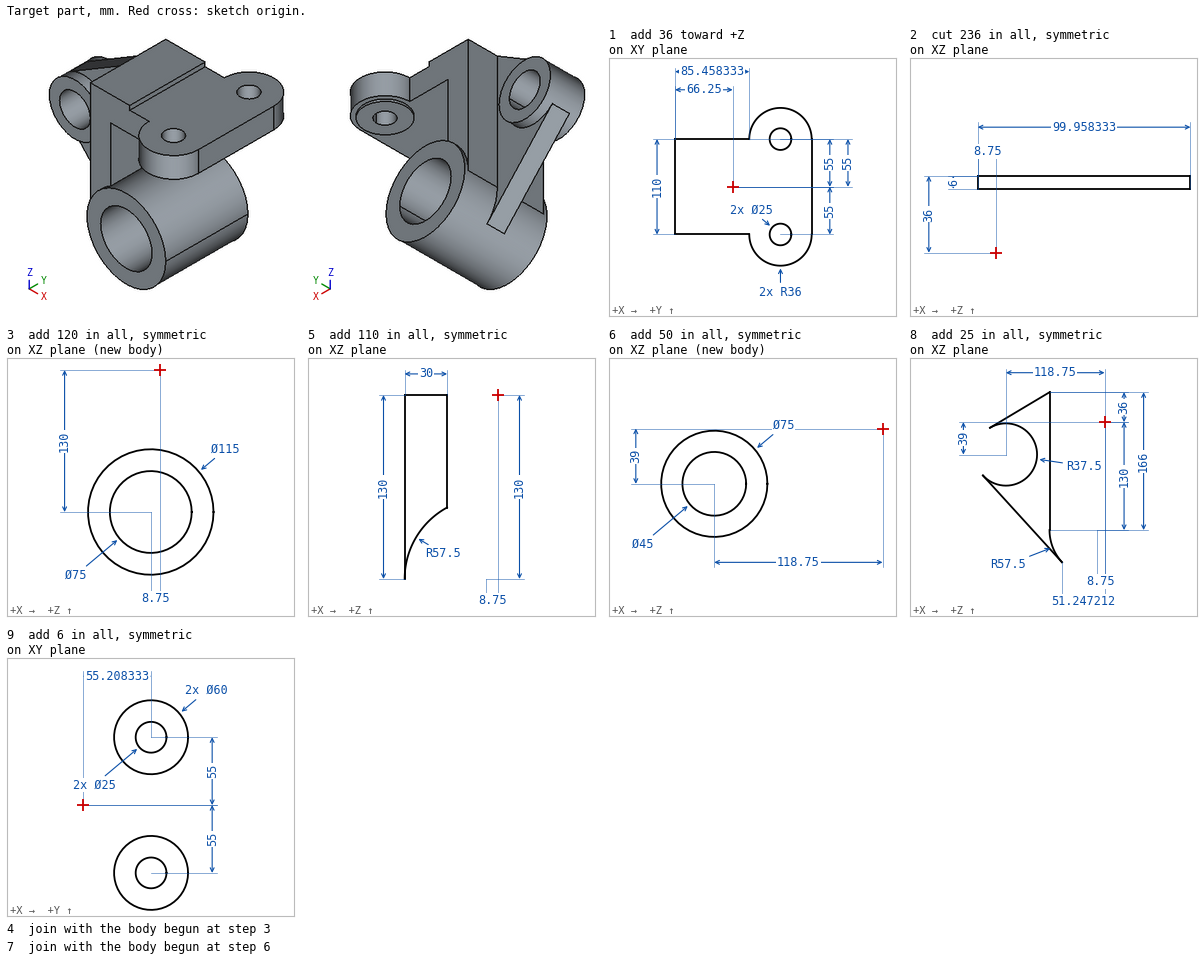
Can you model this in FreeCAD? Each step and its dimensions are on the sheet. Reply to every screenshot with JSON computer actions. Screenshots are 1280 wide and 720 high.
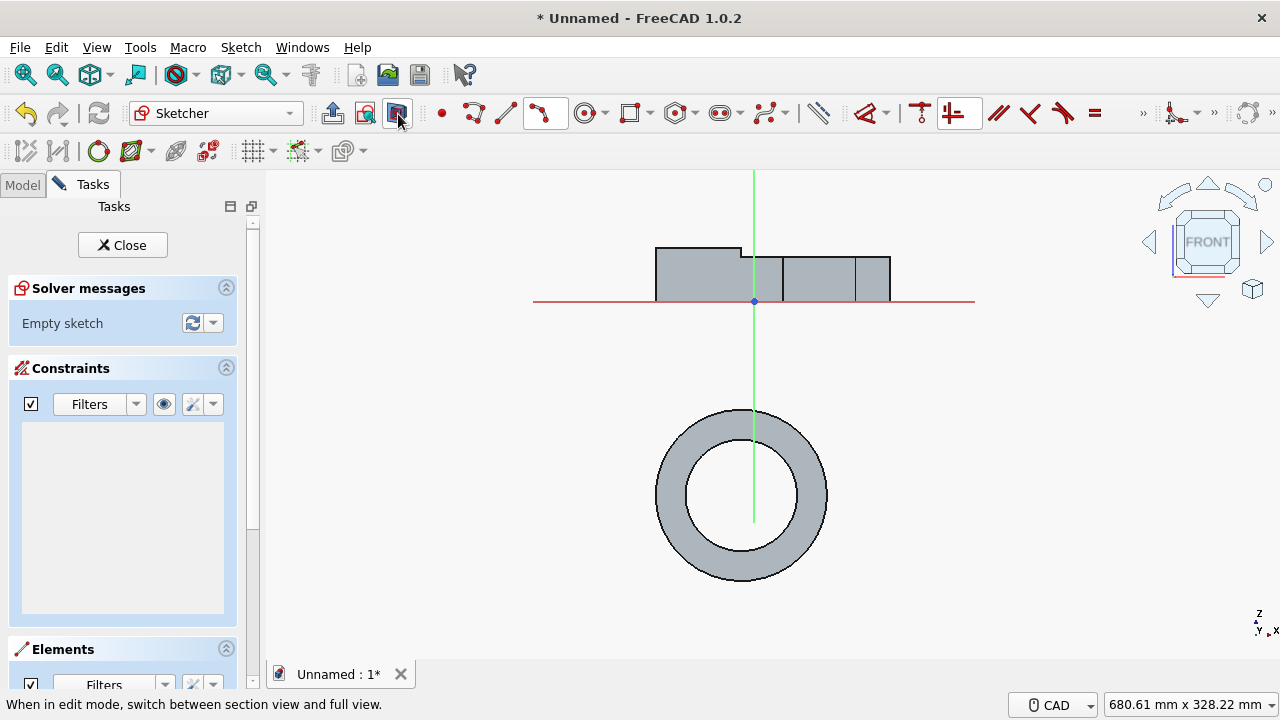
{"action": "scroll", "coordinate": [706, 366], "scroll_direction": "up", "scroll_amount": 2}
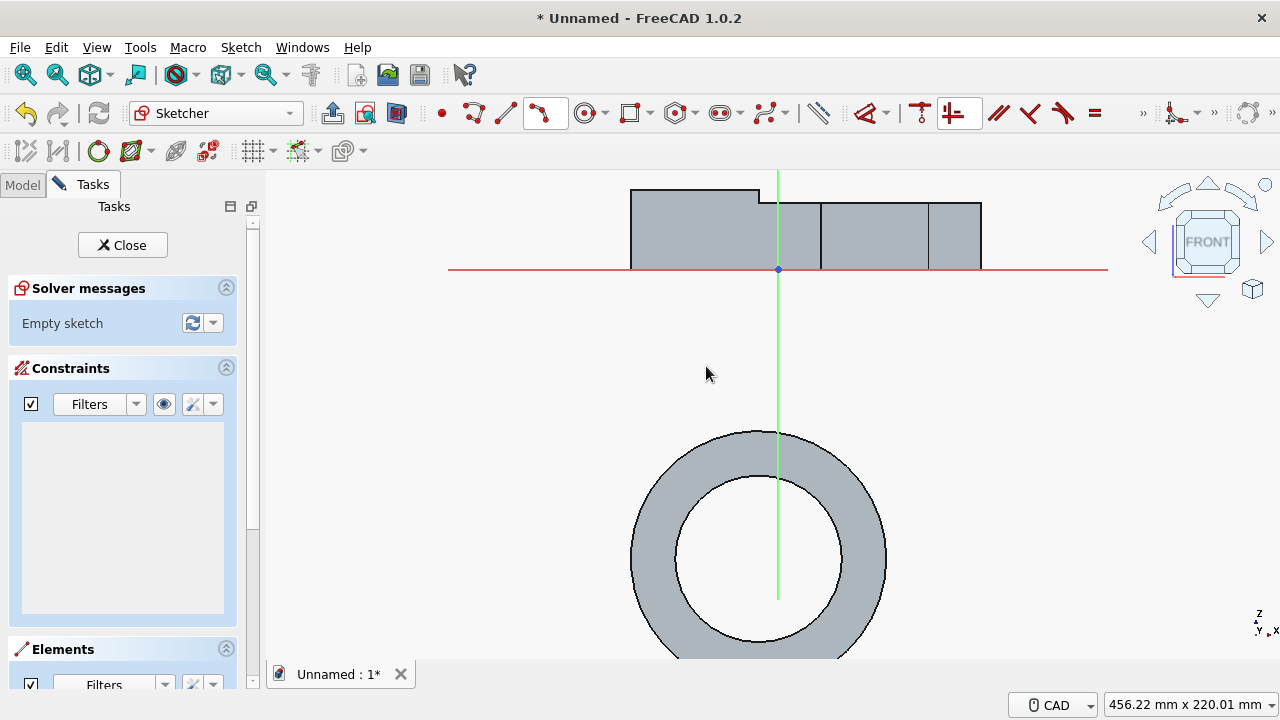
{"action": "left_click", "coordinate": [474, 114]}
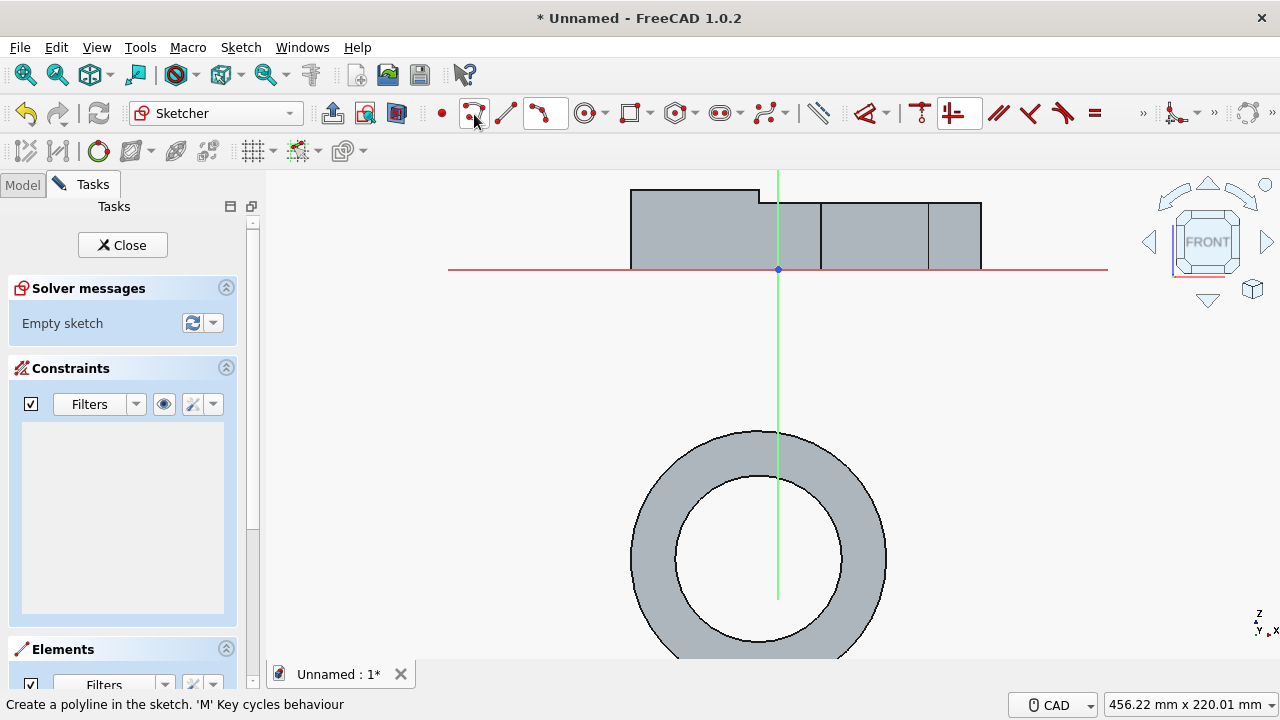
{"action": "left_click", "coordinate": [631, 559]}
{"action": "left_click", "coordinate": [631, 270]}
{"action": "left_click", "coordinate": [697, 279]}
{"action": "left_click", "coordinate": [697, 447]}
{"action": "right_click", "coordinate": [697, 447]}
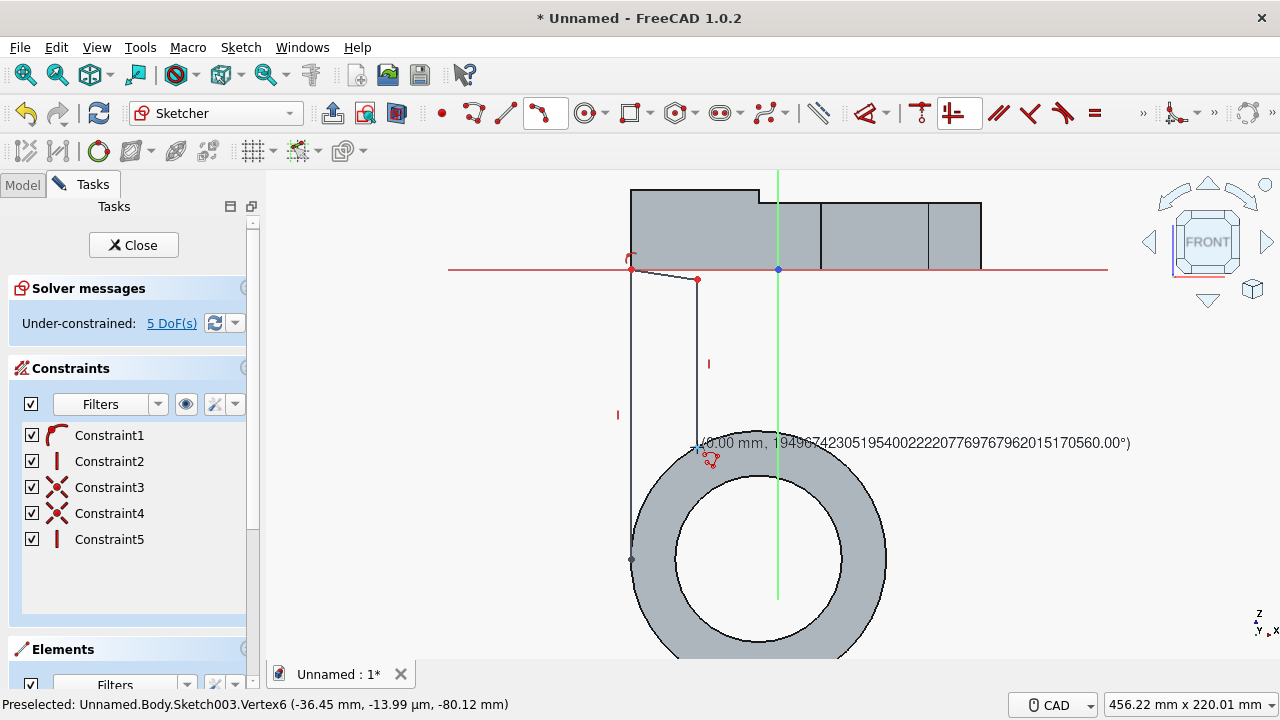
{"action": "left_click", "coordinate": [540, 114]}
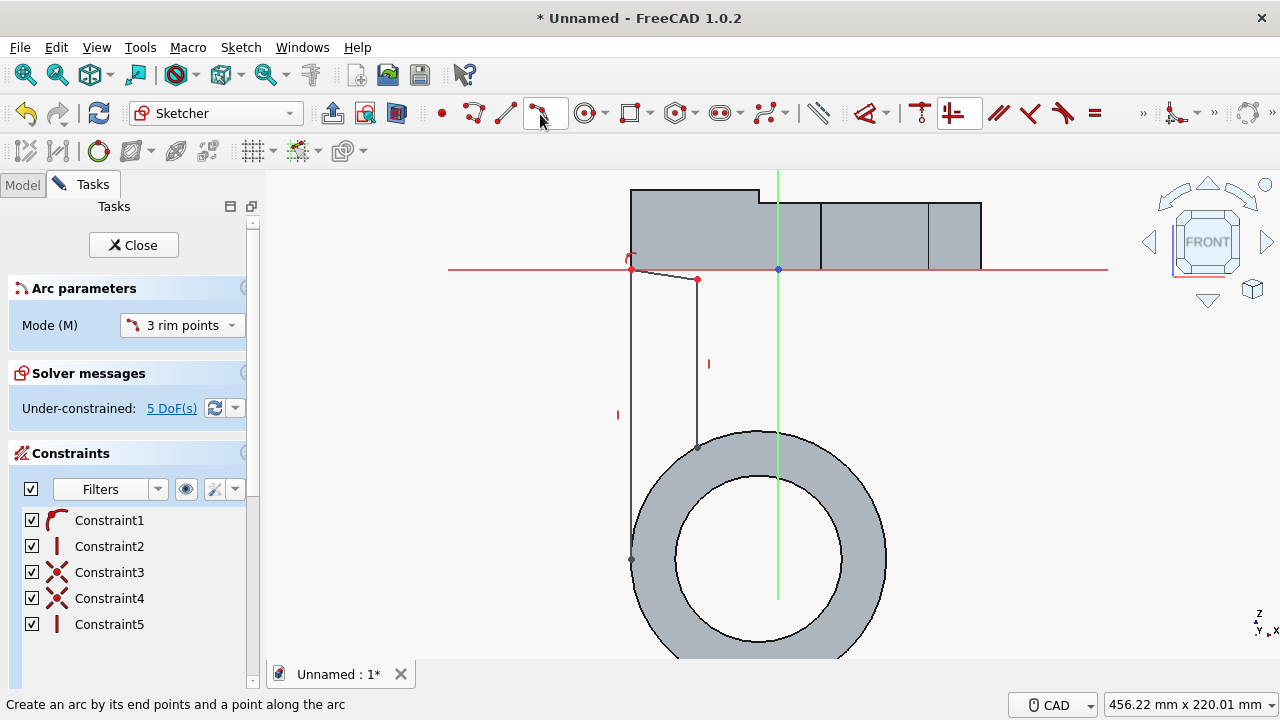
{"action": "left_click", "coordinate": [697, 448]}
{"action": "left_click", "coordinate": [631, 560]}
{"action": "left_click", "coordinate": [649, 494]}
{"action": "key", "text": "Escape"}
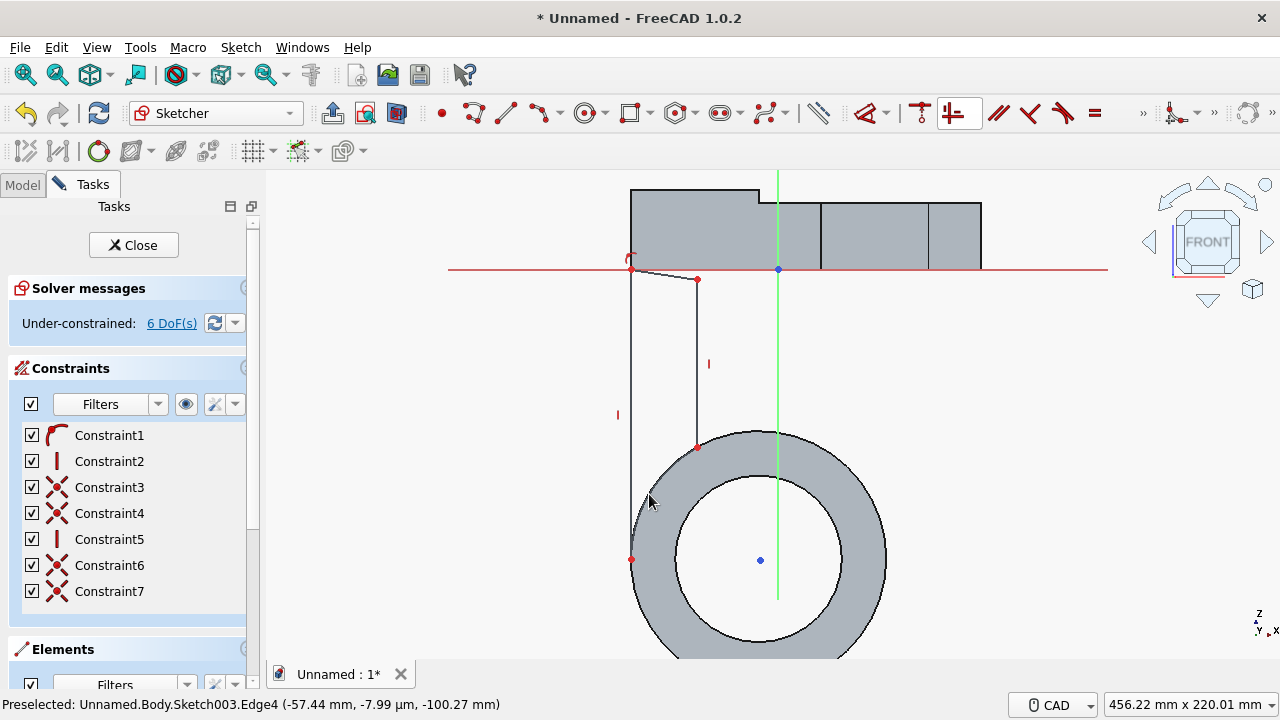
{"action": "left_click", "coordinate": [651, 273]}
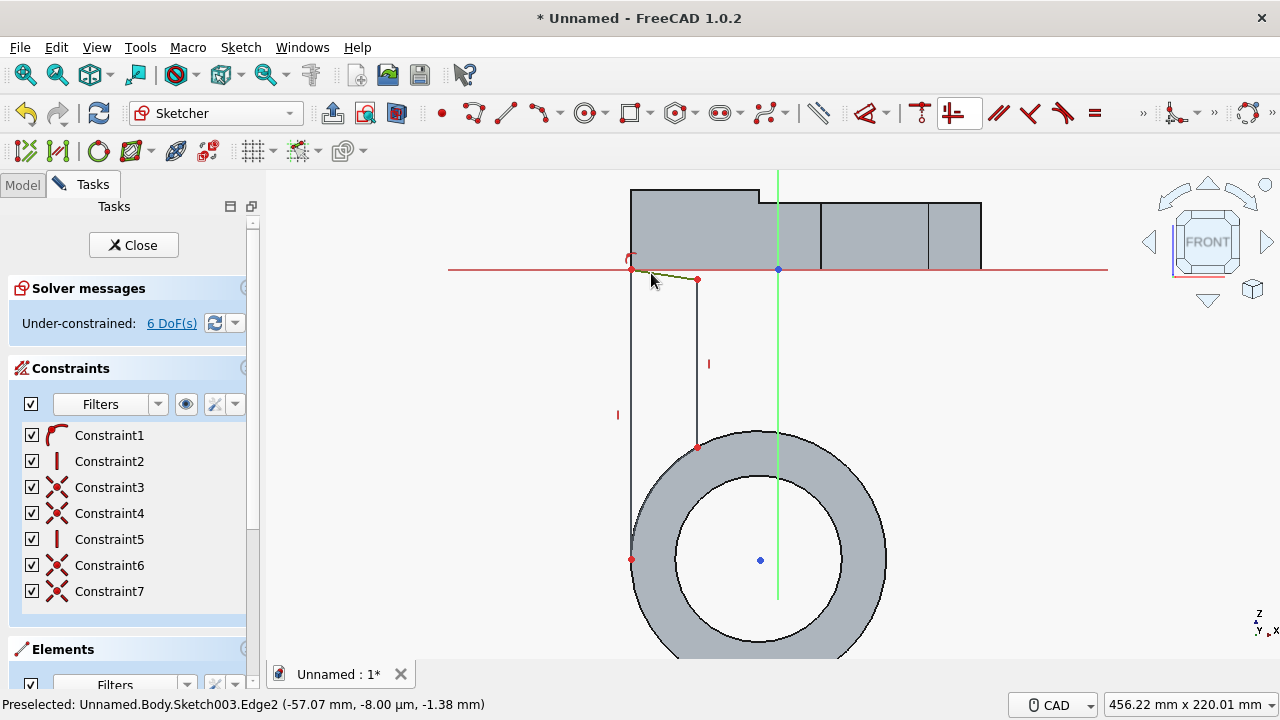
{"action": "left_click", "coordinate": [976, 114]}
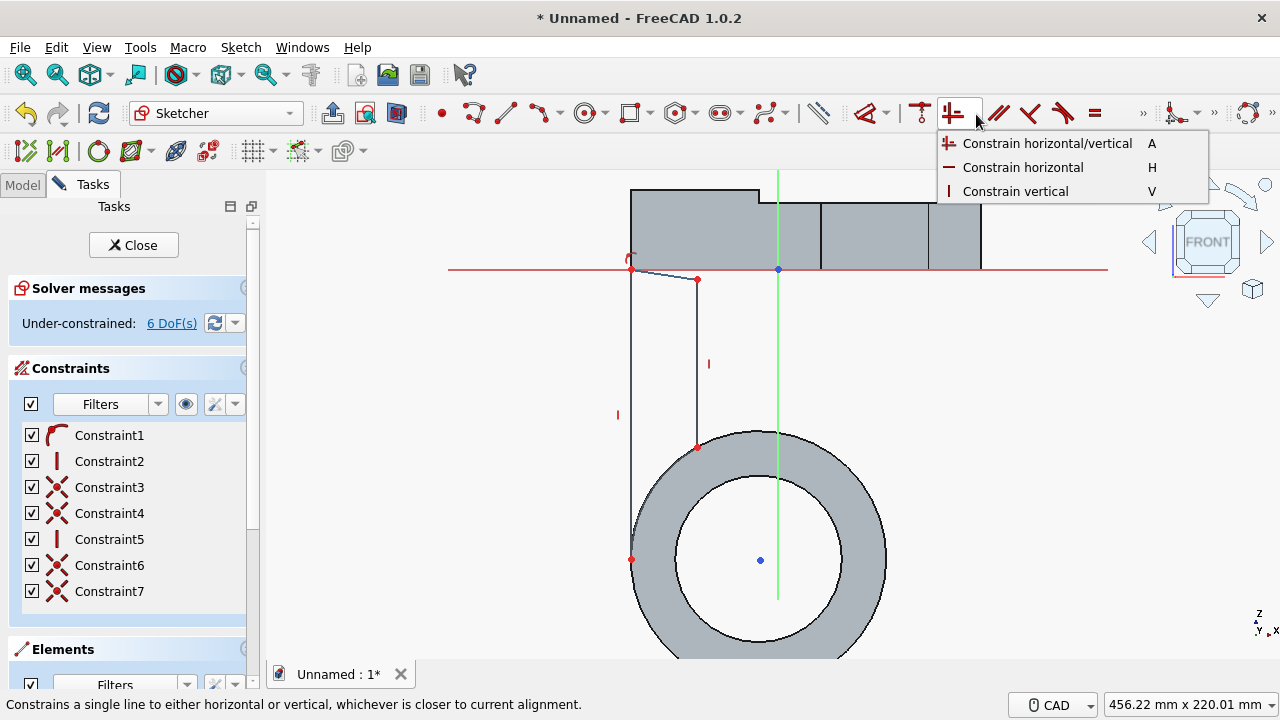
{"action": "left_click", "coordinate": [1073, 167]}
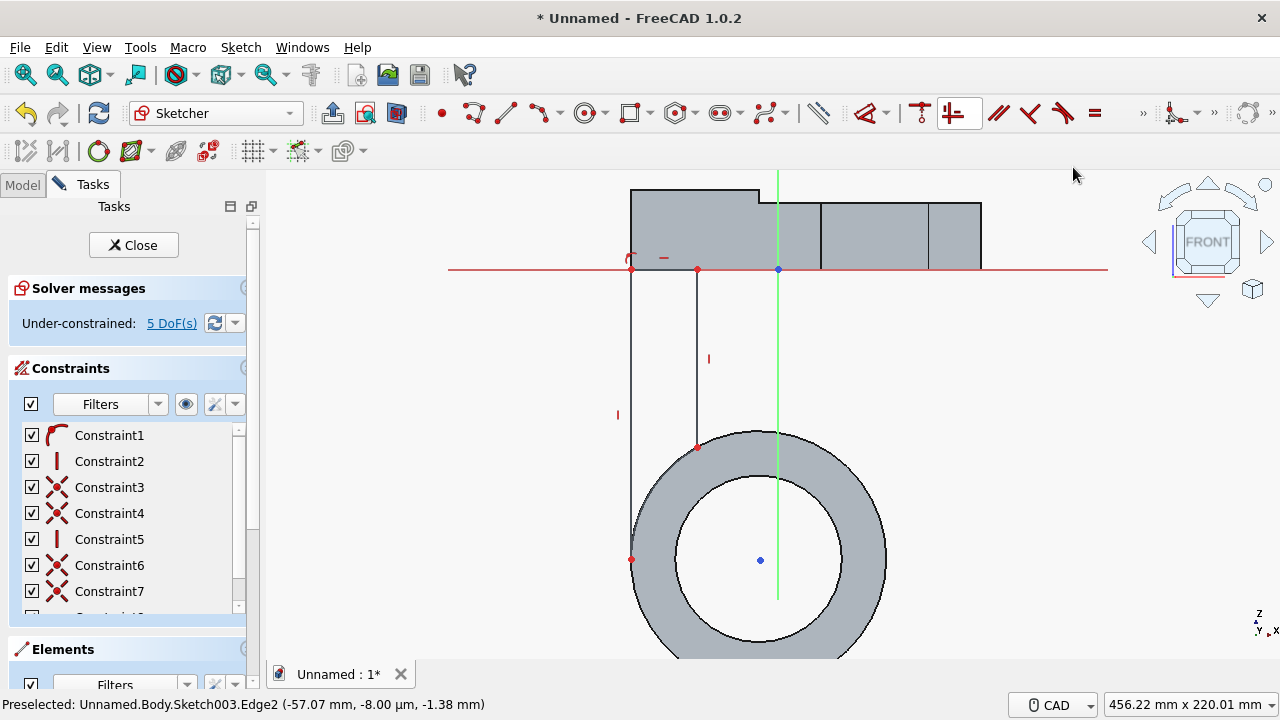
{"action": "left_click", "coordinate": [866, 114]}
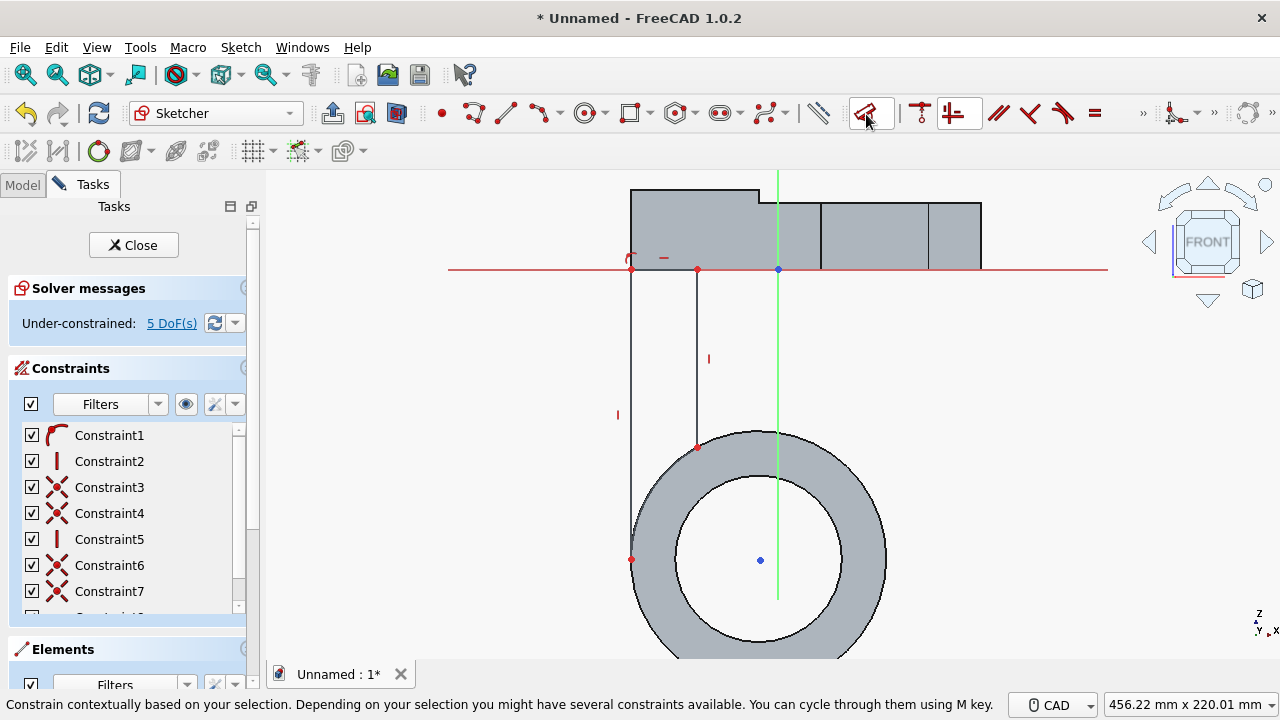
{"action": "left_click", "coordinate": [665, 473]}
{"action": "left_click", "coordinate": [604, 522]}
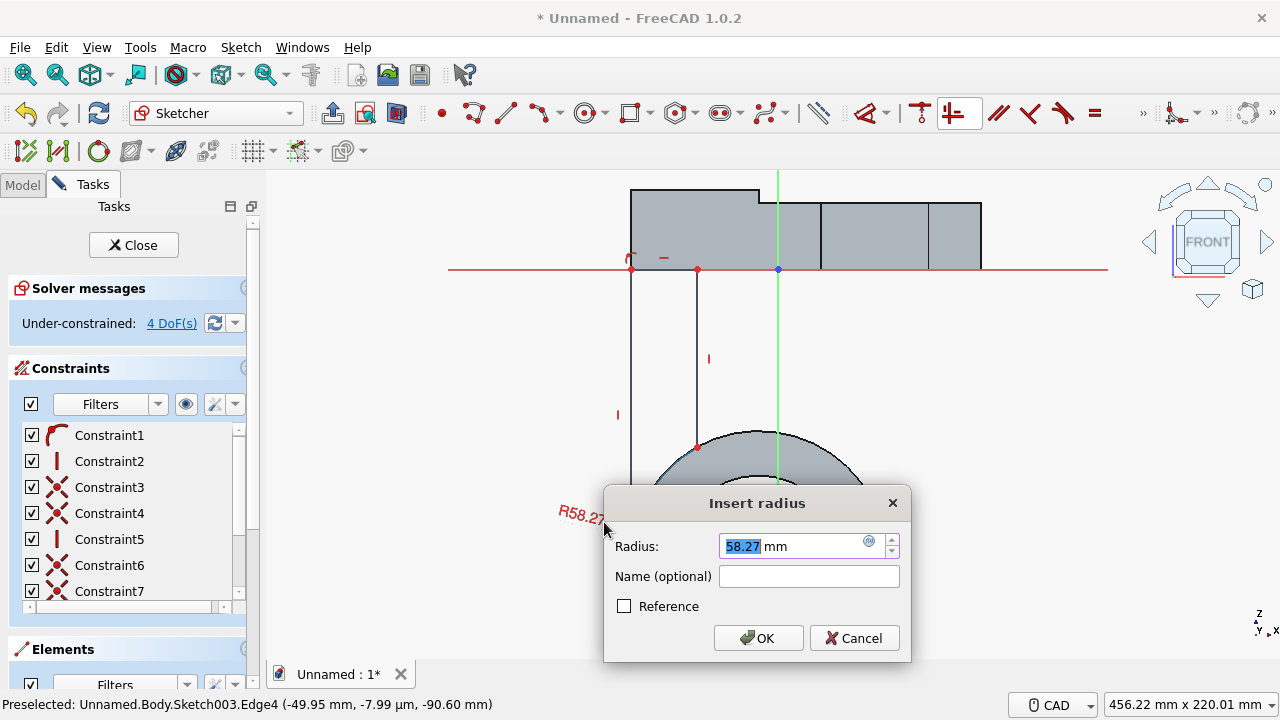
{"action": "type", "text": "57.5"}
{"action": "key", "text": "Return"}